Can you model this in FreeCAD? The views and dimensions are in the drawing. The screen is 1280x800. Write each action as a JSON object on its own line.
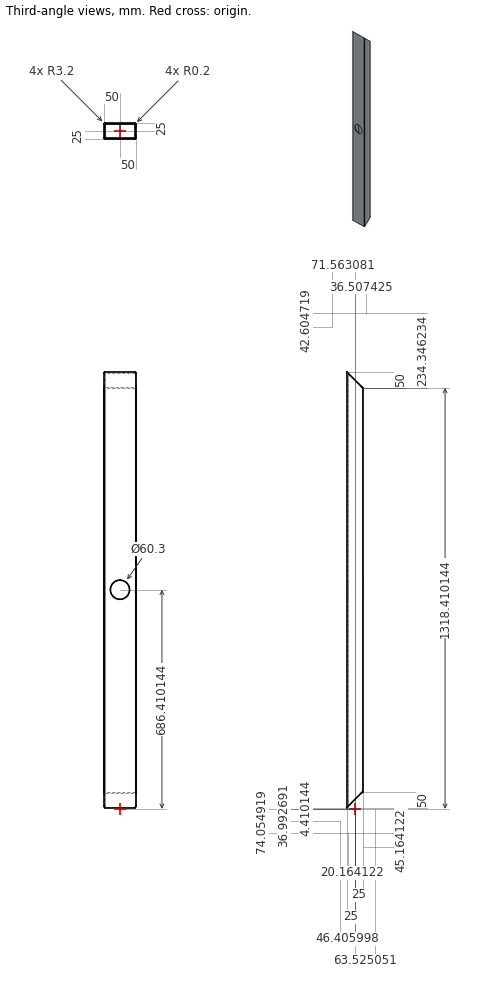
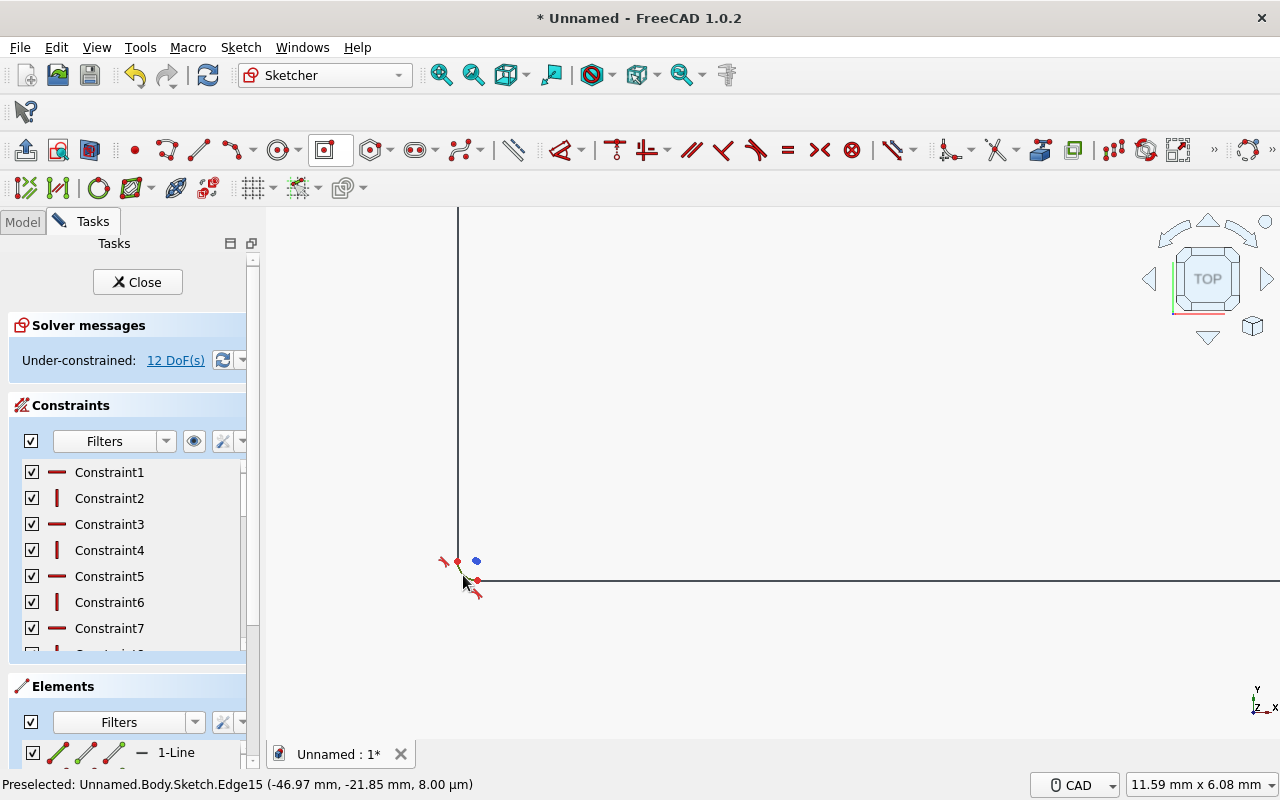
{"action": "key", "text": "c"}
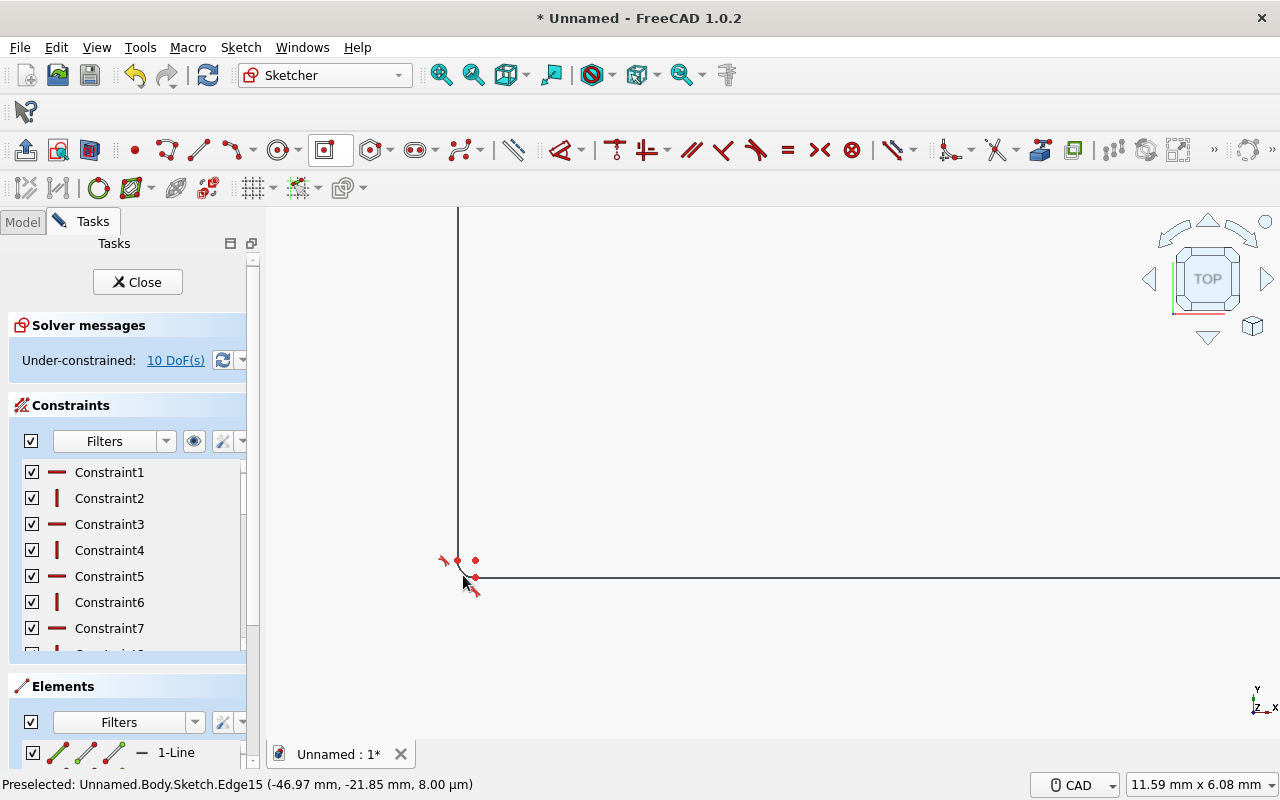
{"action": "scroll", "coordinate": [454, 590], "scroll_direction": "down", "scroll_amount": 14}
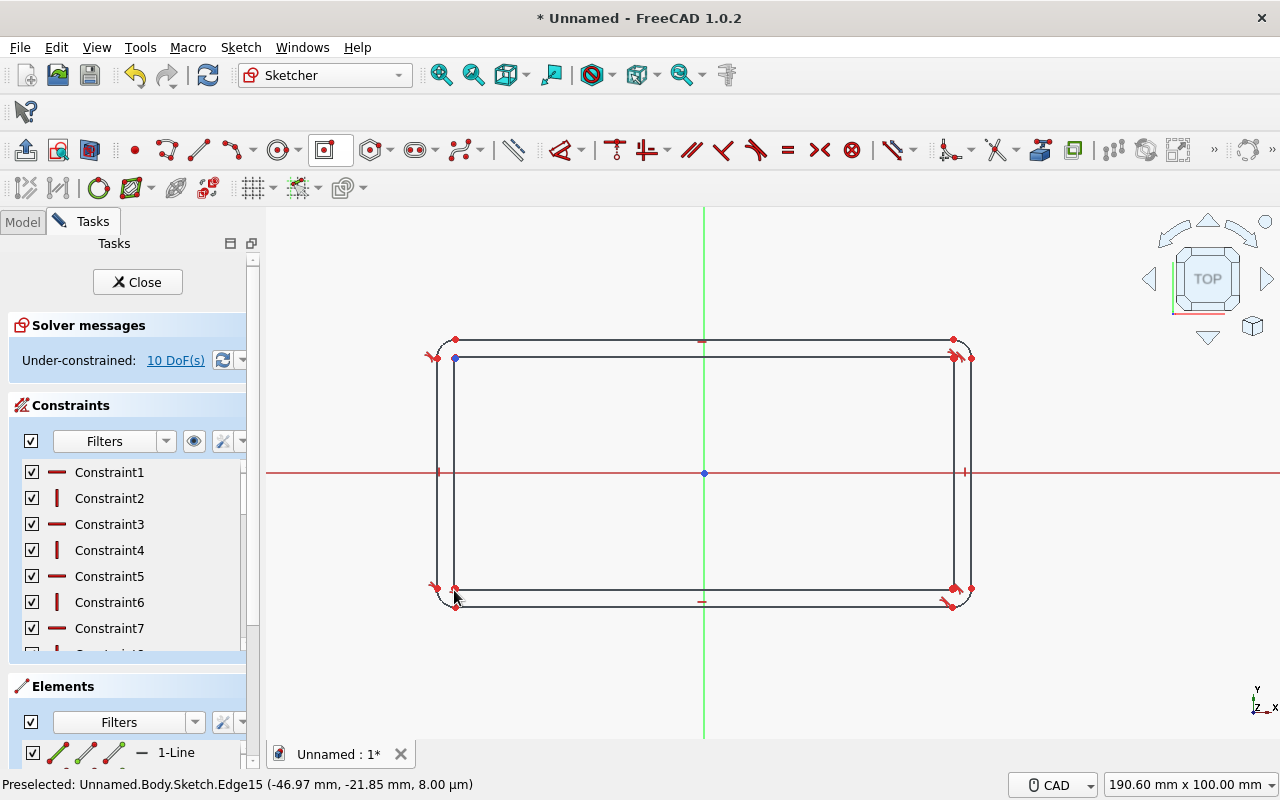
{"action": "scroll", "coordinate": [447, 342], "scroll_direction": "up", "scroll_amount": 3}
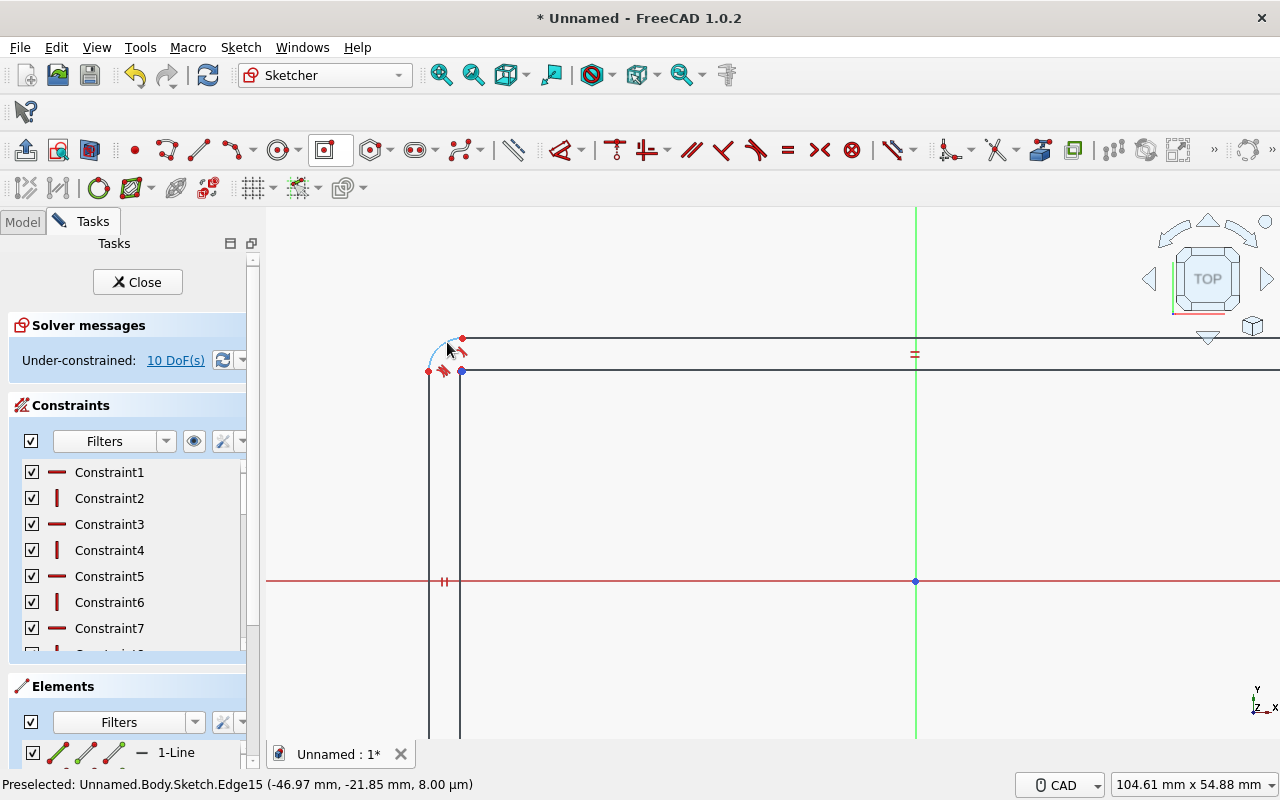
{"action": "left_click", "coordinate": [447, 342]}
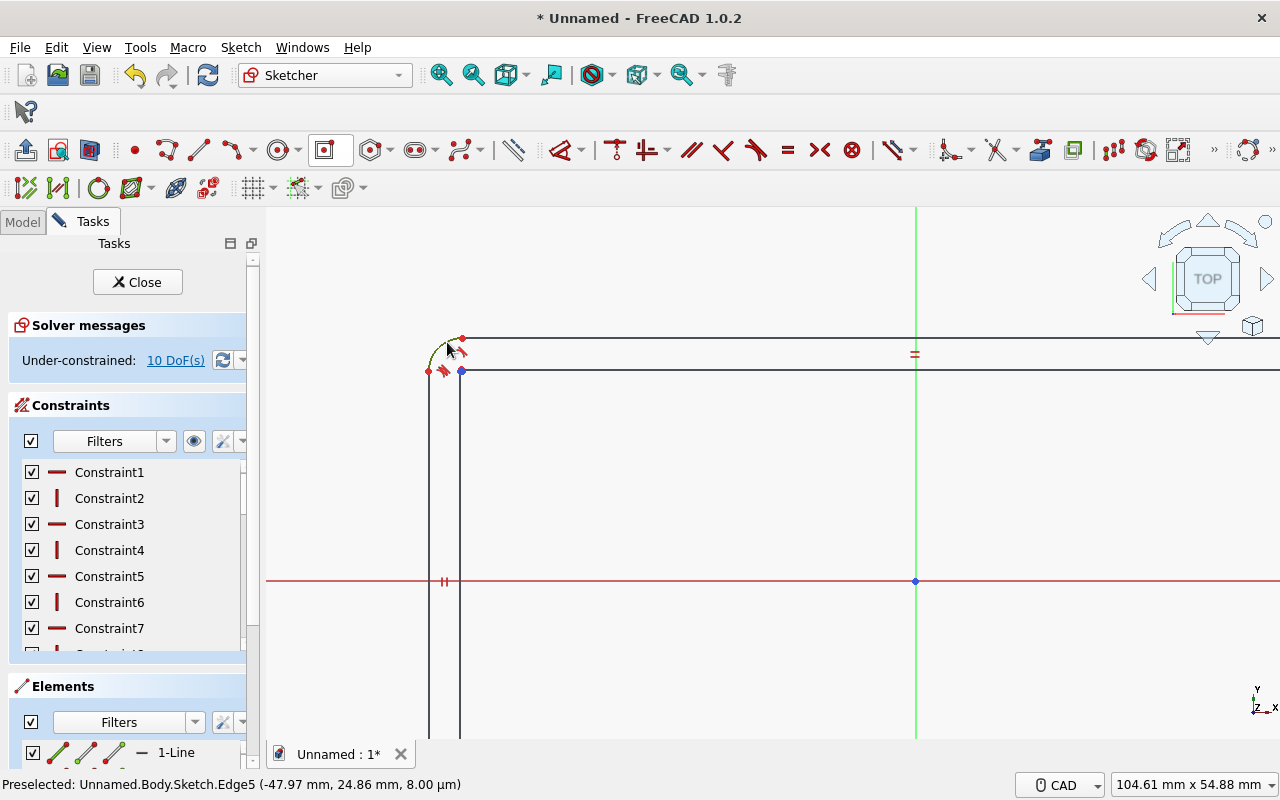
{"action": "scroll", "coordinate": [447, 342], "scroll_direction": "down", "scroll_amount": 3}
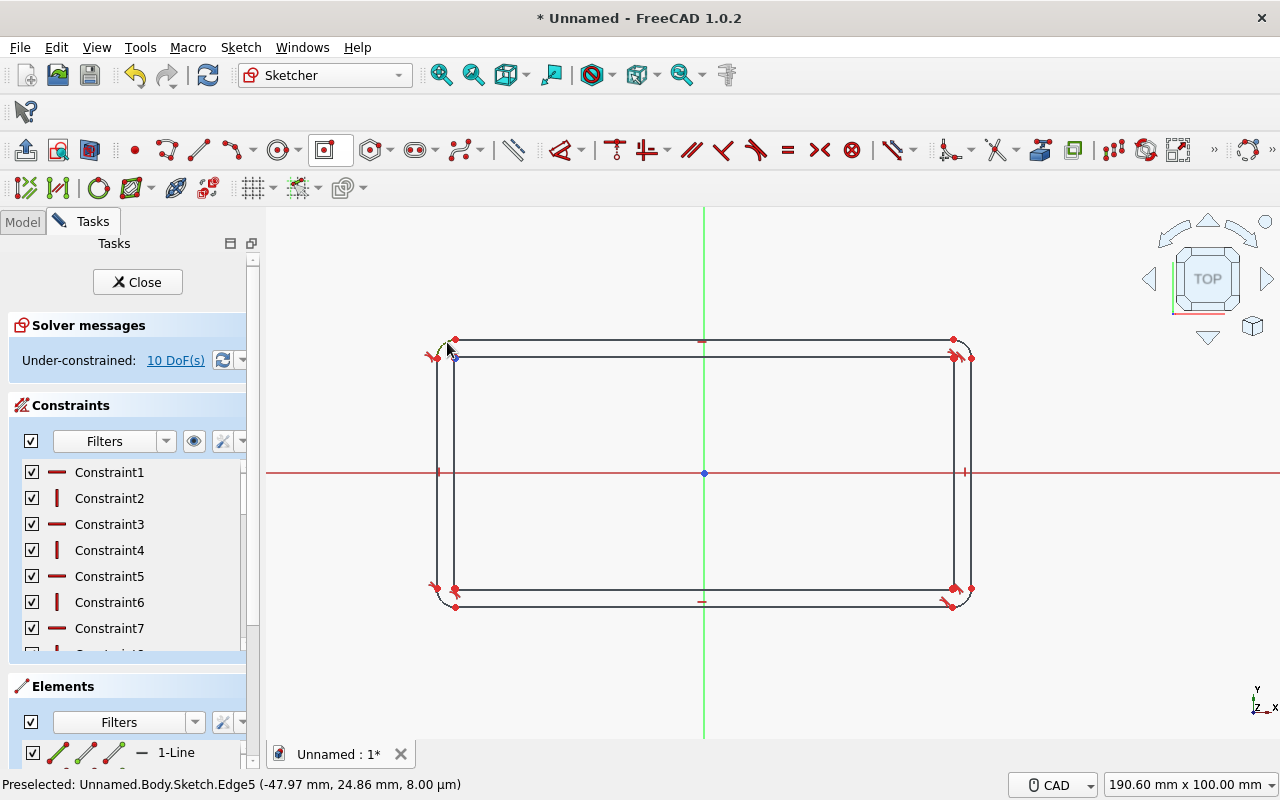
{"action": "scroll", "coordinate": [439, 597], "scroll_direction": "up", "scroll_amount": 3}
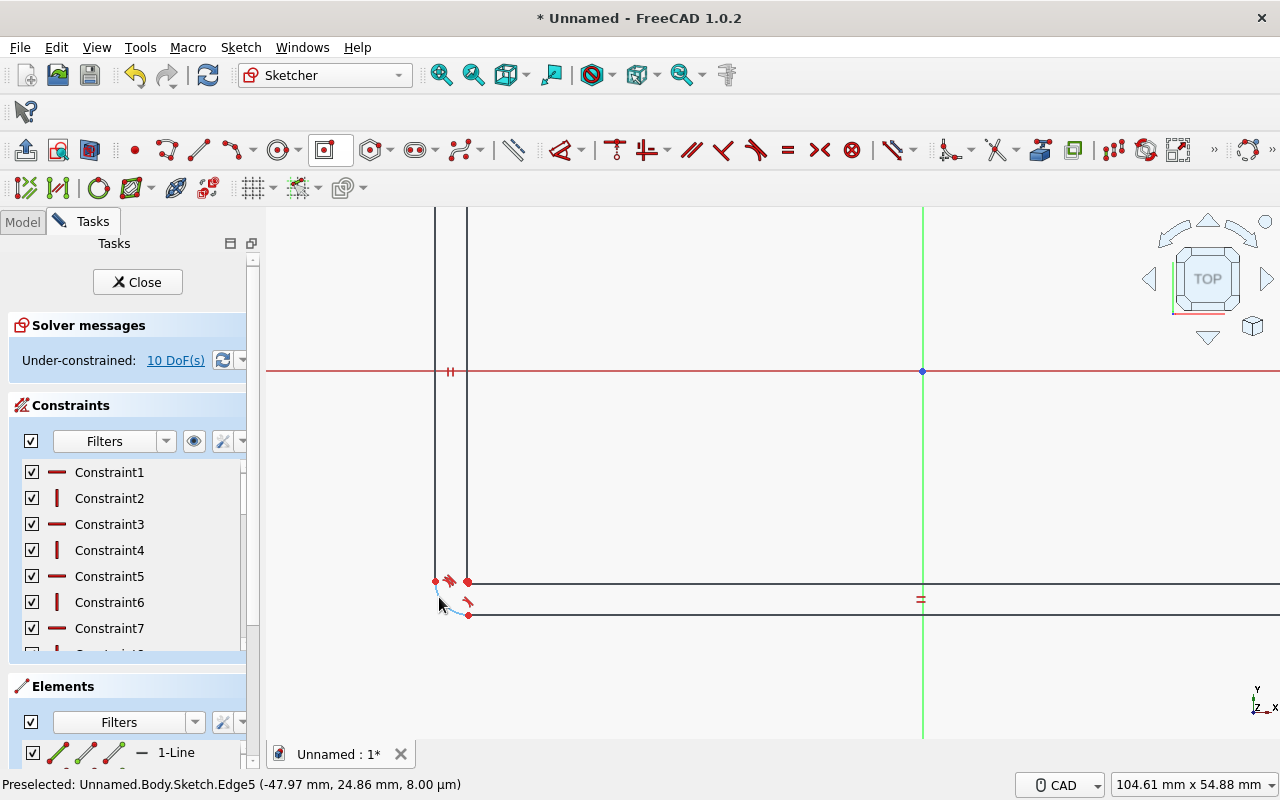
{"action": "left_click", "coordinate": [439, 597]}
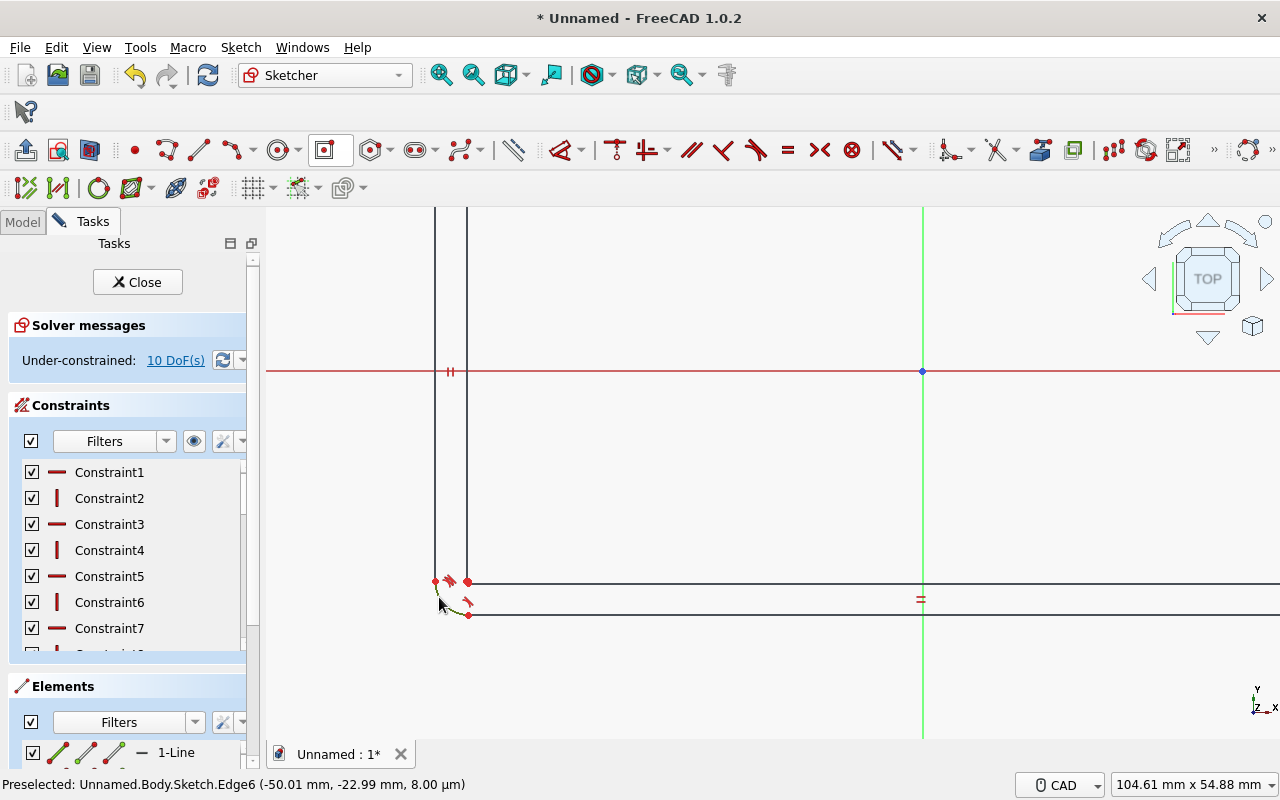
{"action": "scroll", "coordinate": [439, 597], "scroll_direction": "down", "scroll_amount": 3}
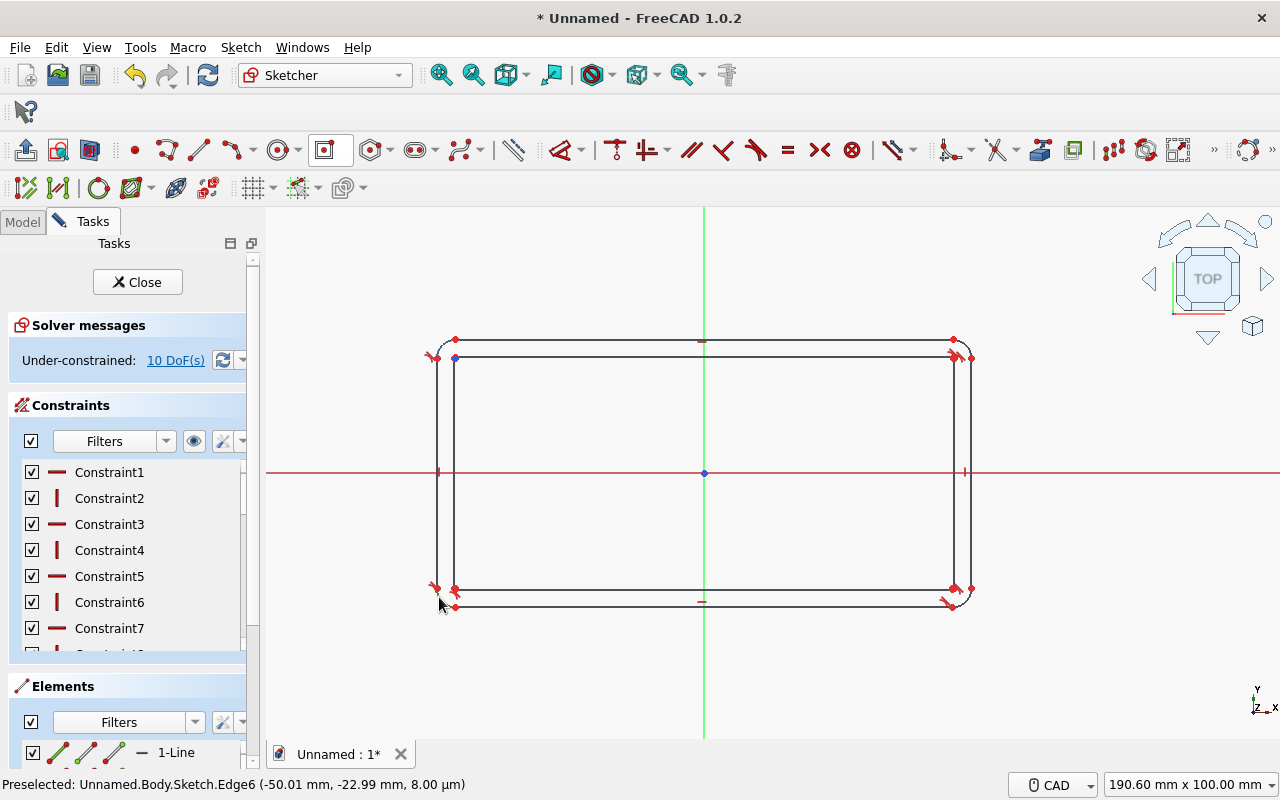
{"action": "scroll", "coordinate": [961, 605], "scroll_direction": "up", "scroll_amount": 3}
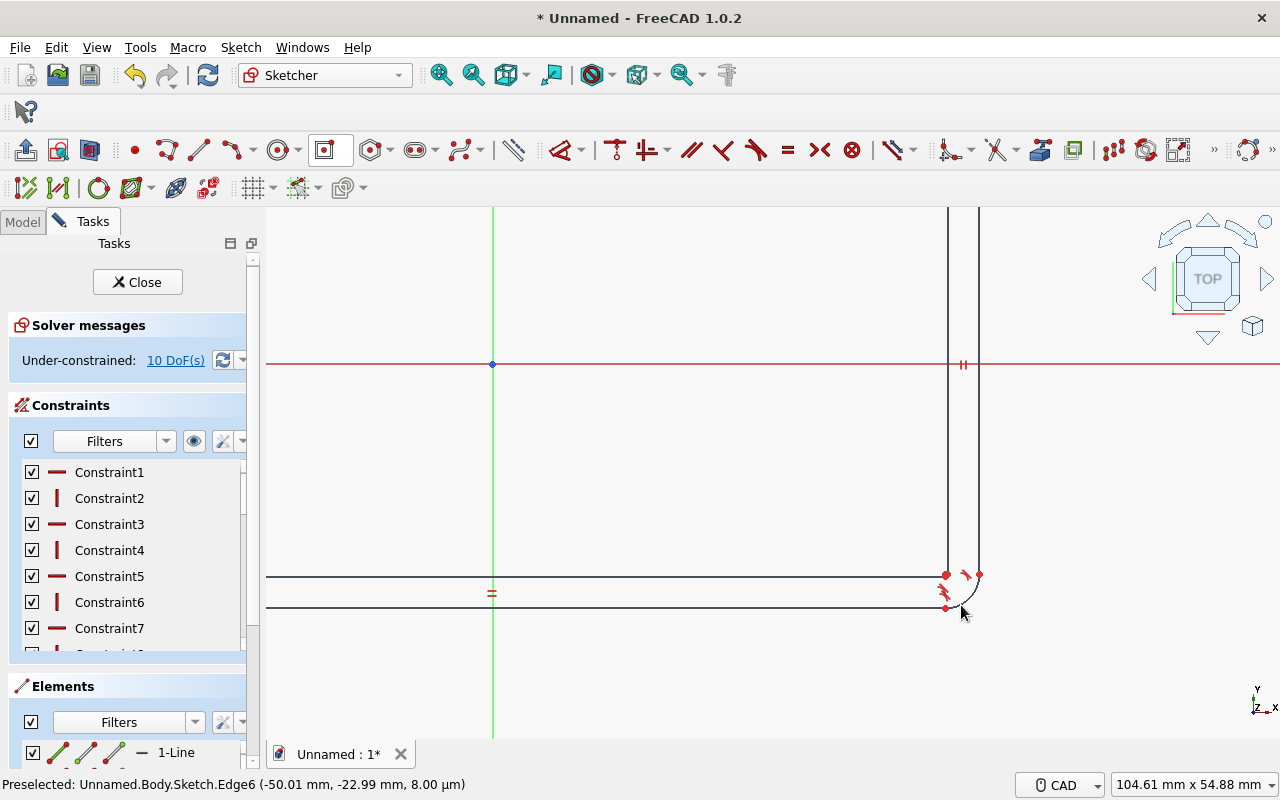
{"action": "left_click", "coordinate": [961, 605]}